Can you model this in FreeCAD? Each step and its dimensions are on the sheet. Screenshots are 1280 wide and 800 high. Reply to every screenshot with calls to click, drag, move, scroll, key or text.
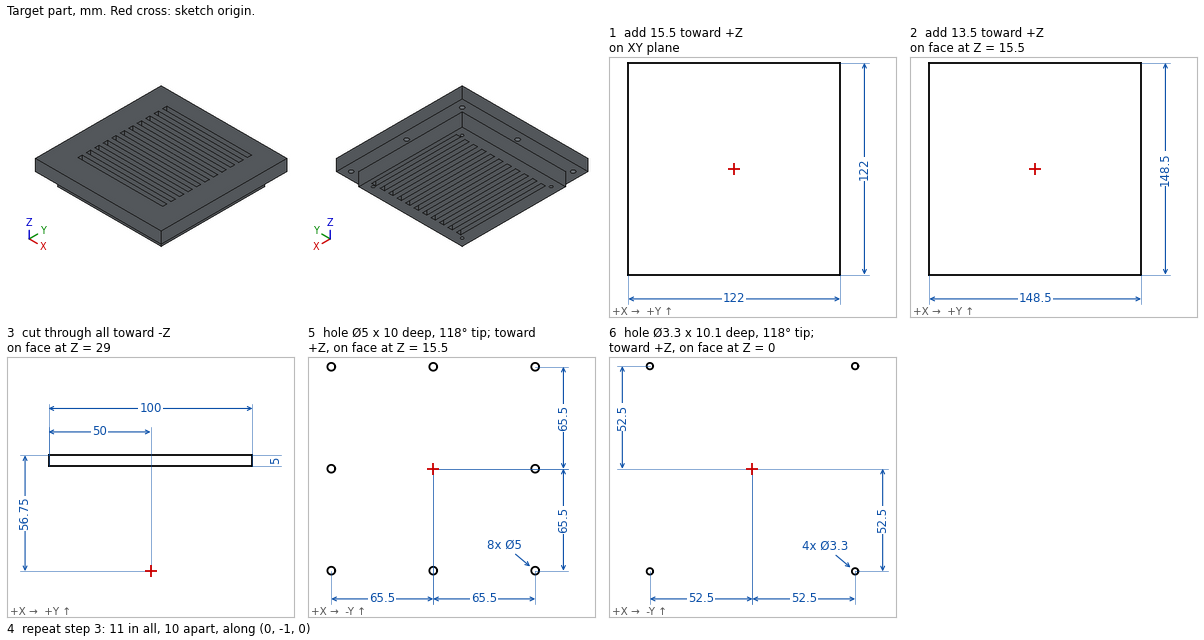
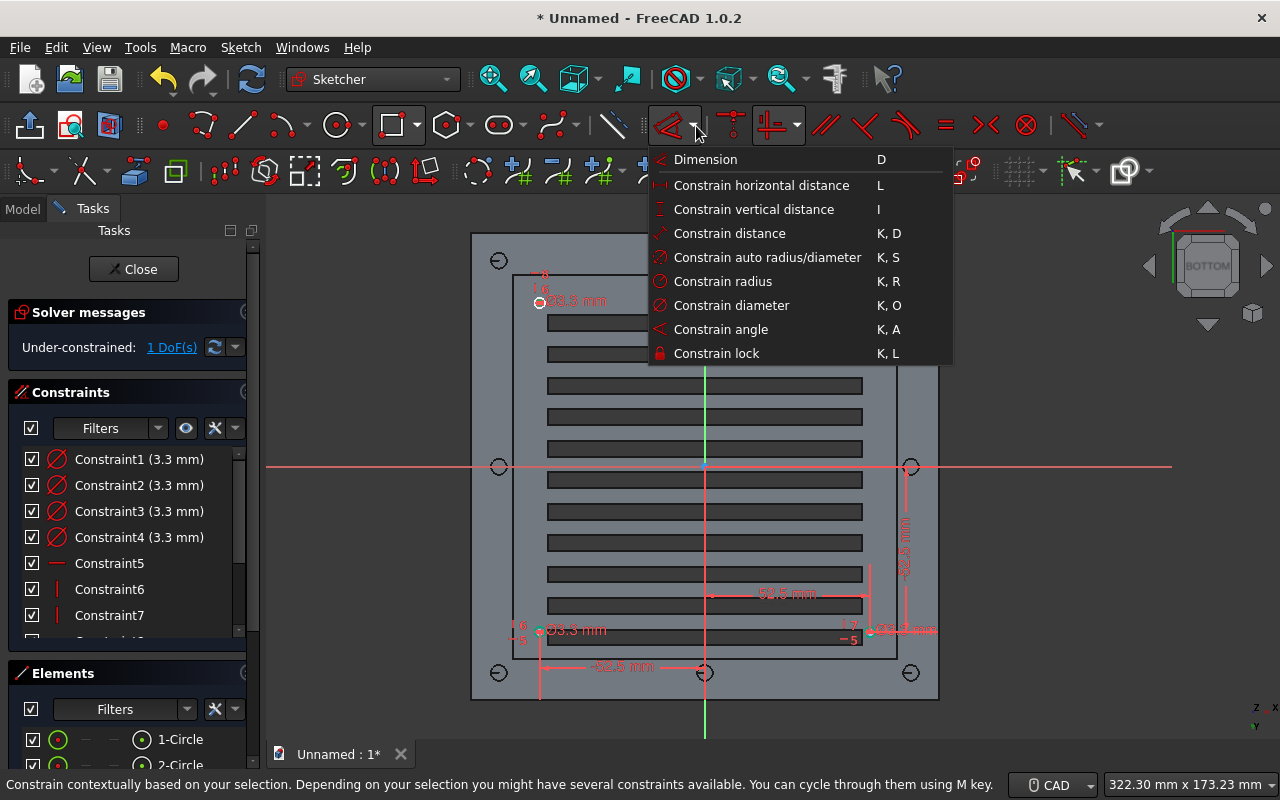
click(801, 209)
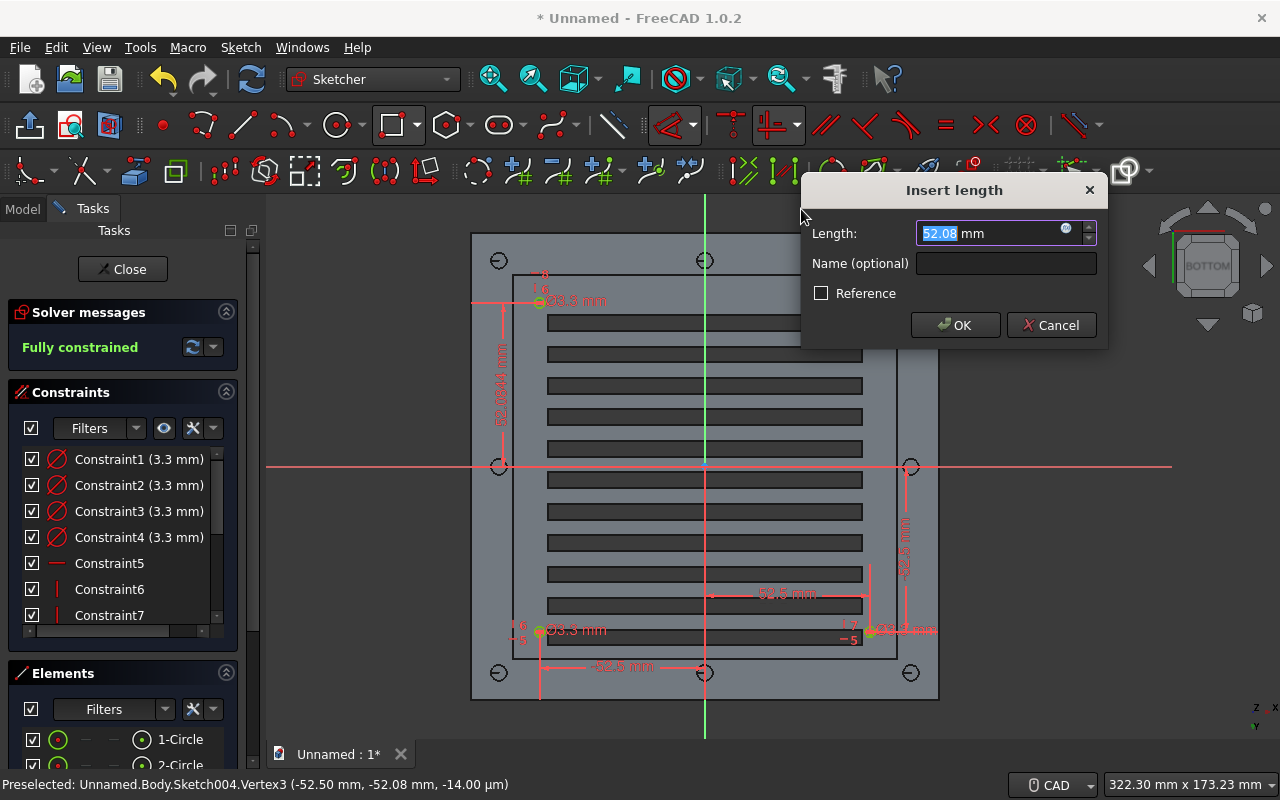
text(52.5)
key(Return)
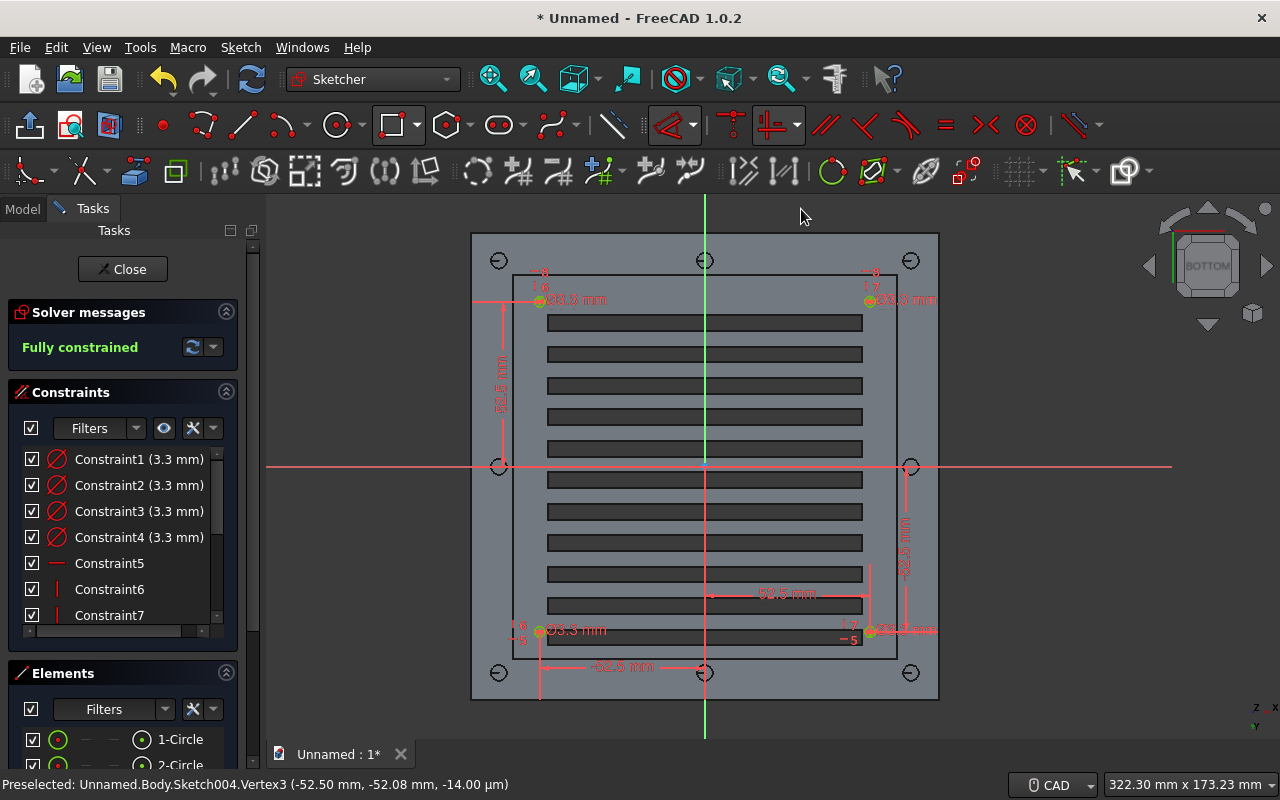
click(123, 269)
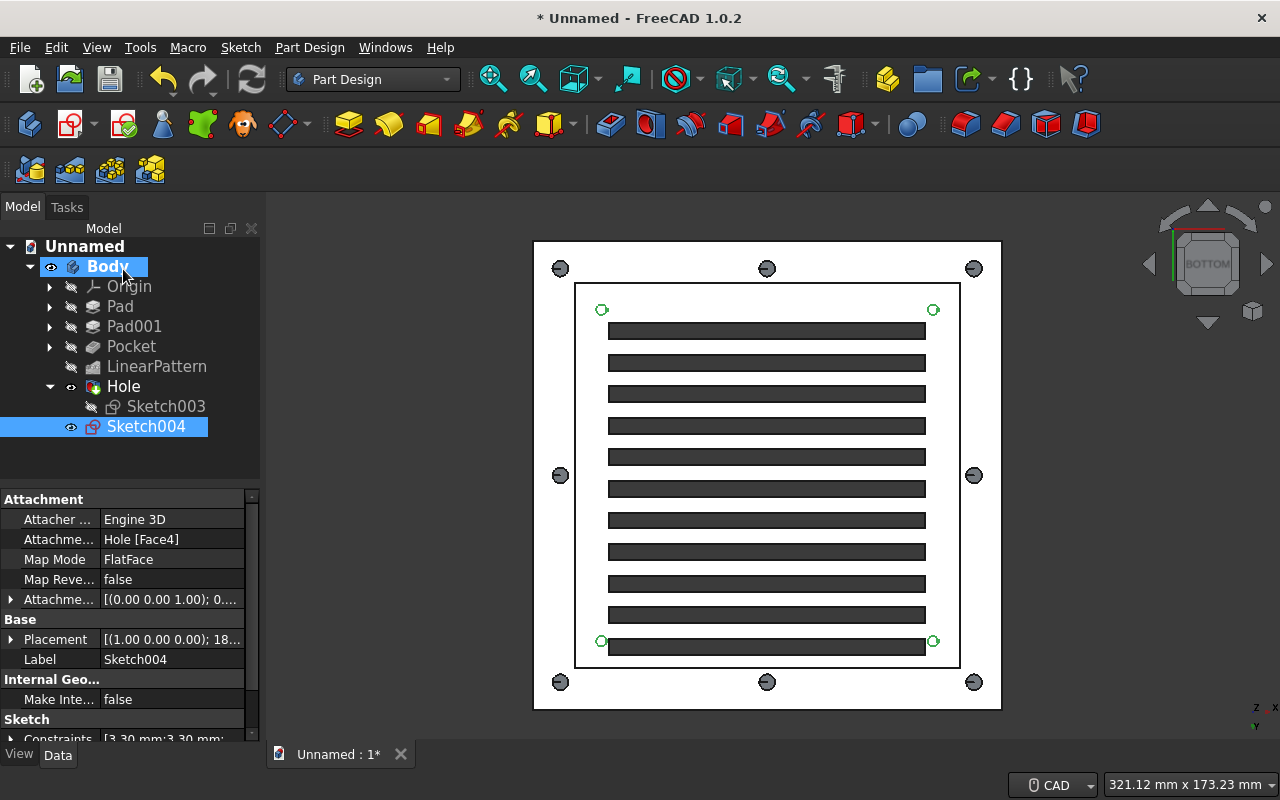
click(652, 124)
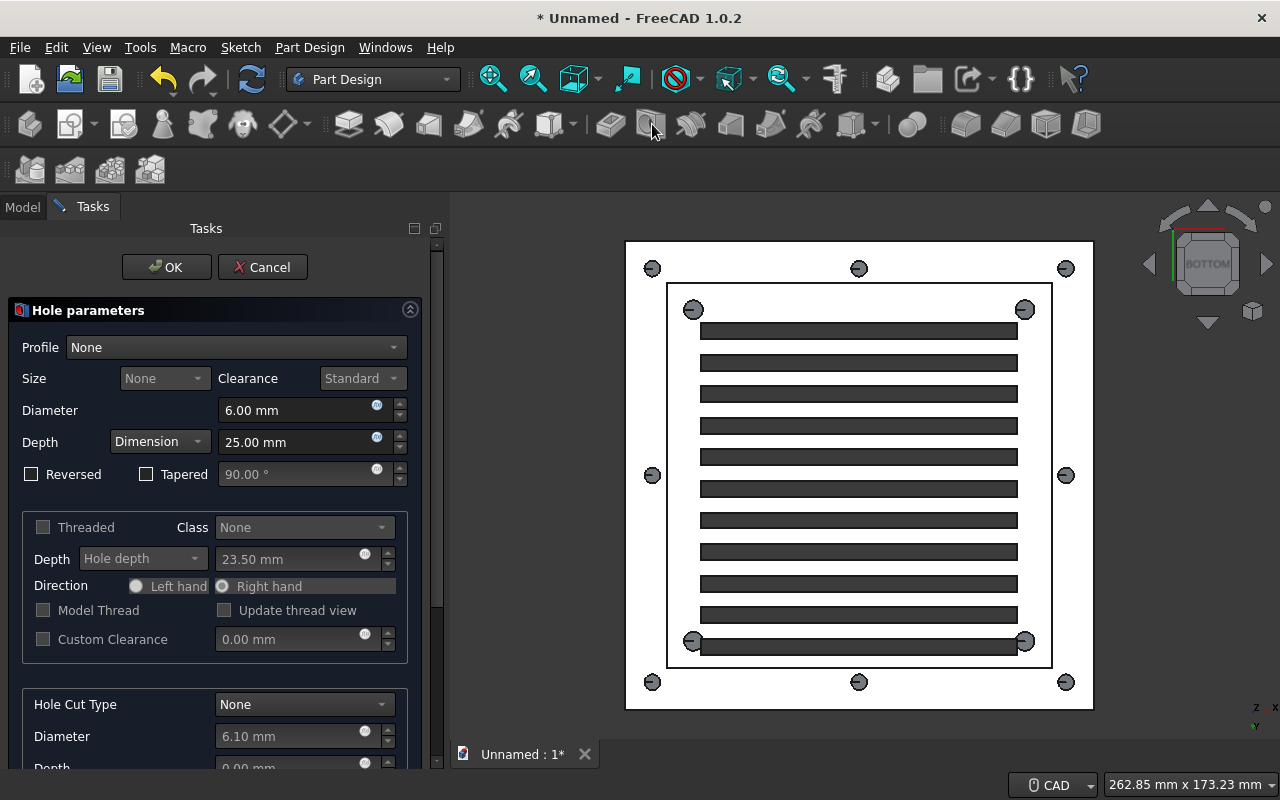
triple_click(305, 410)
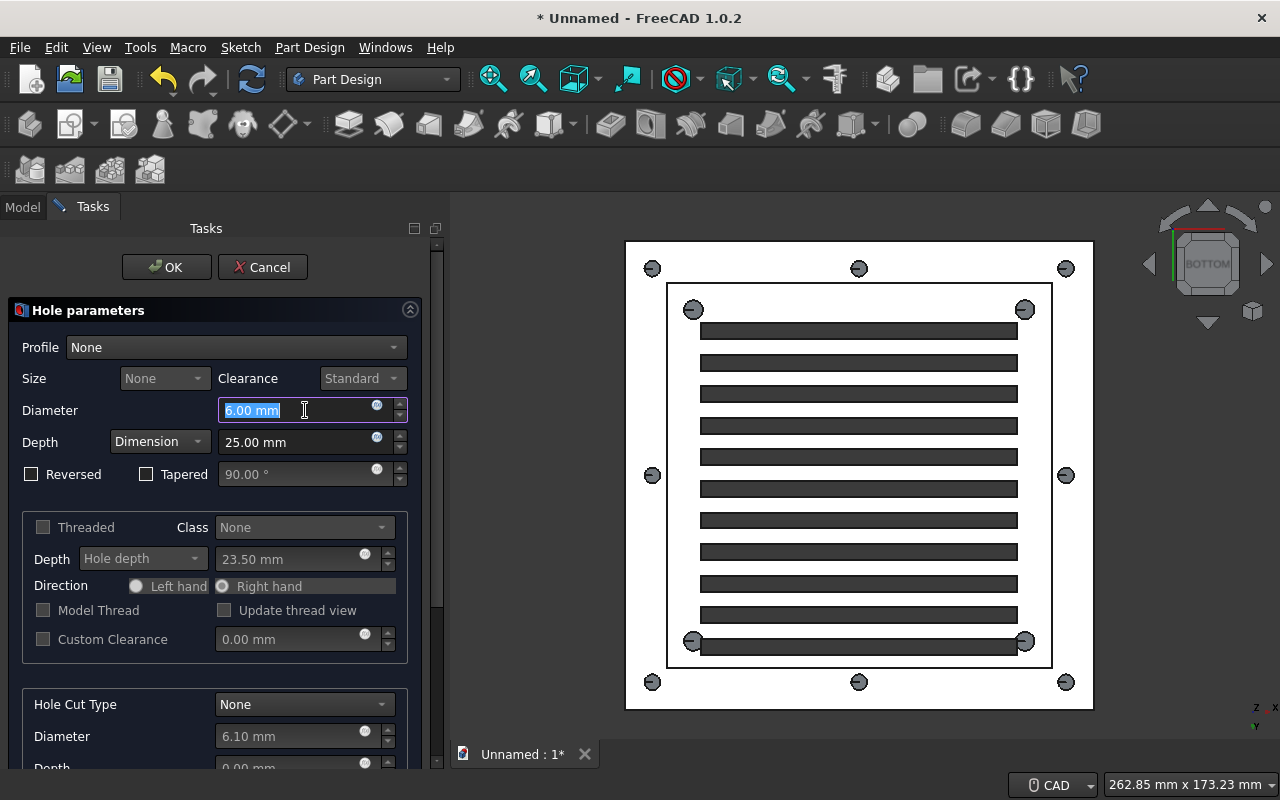
text(3.3)
key(Tab)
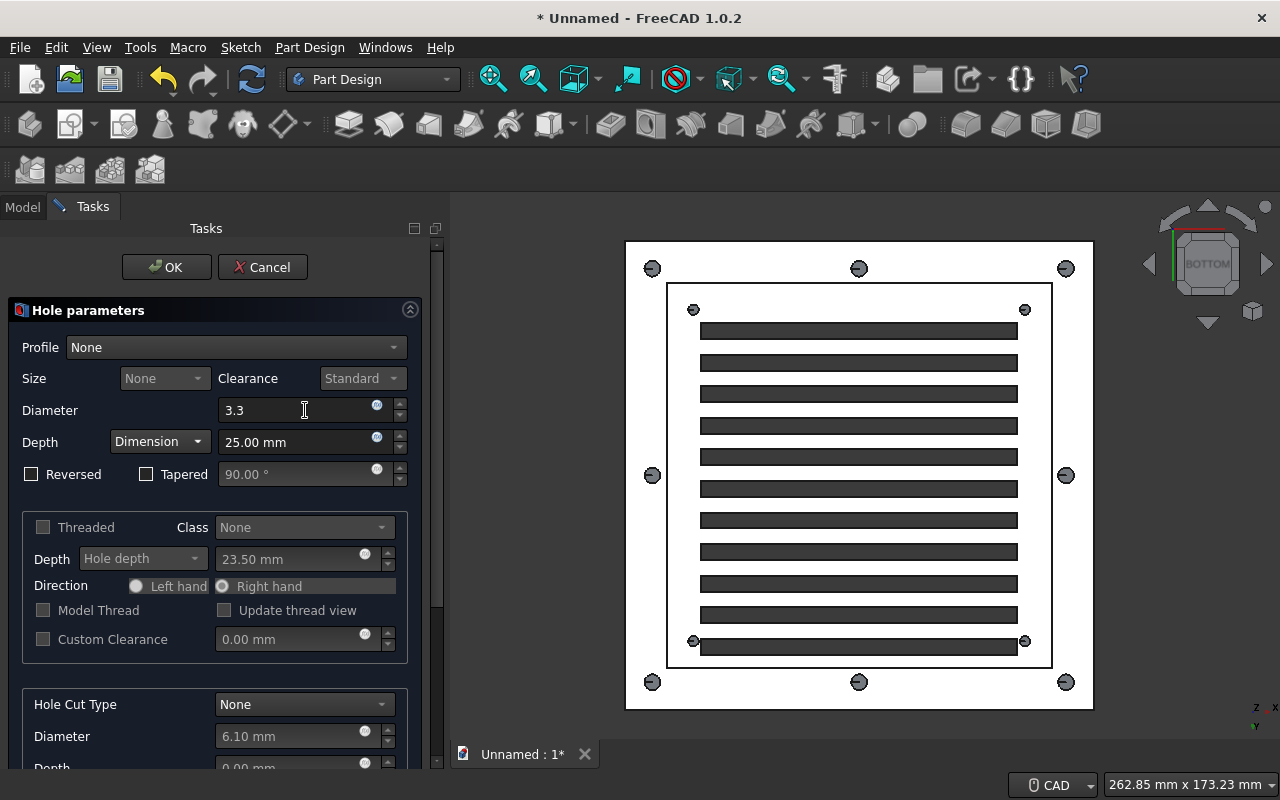
triple_click(305, 442)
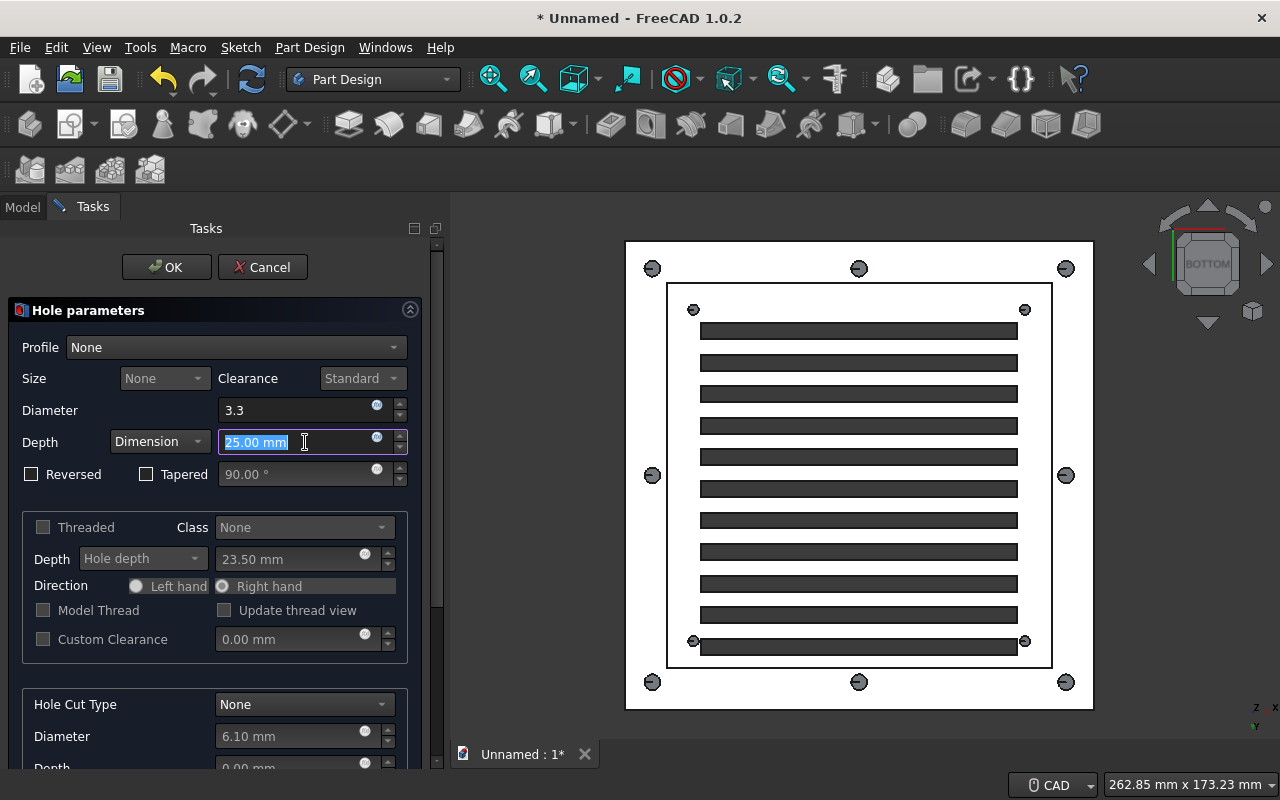
text(10.1)
key(Tab)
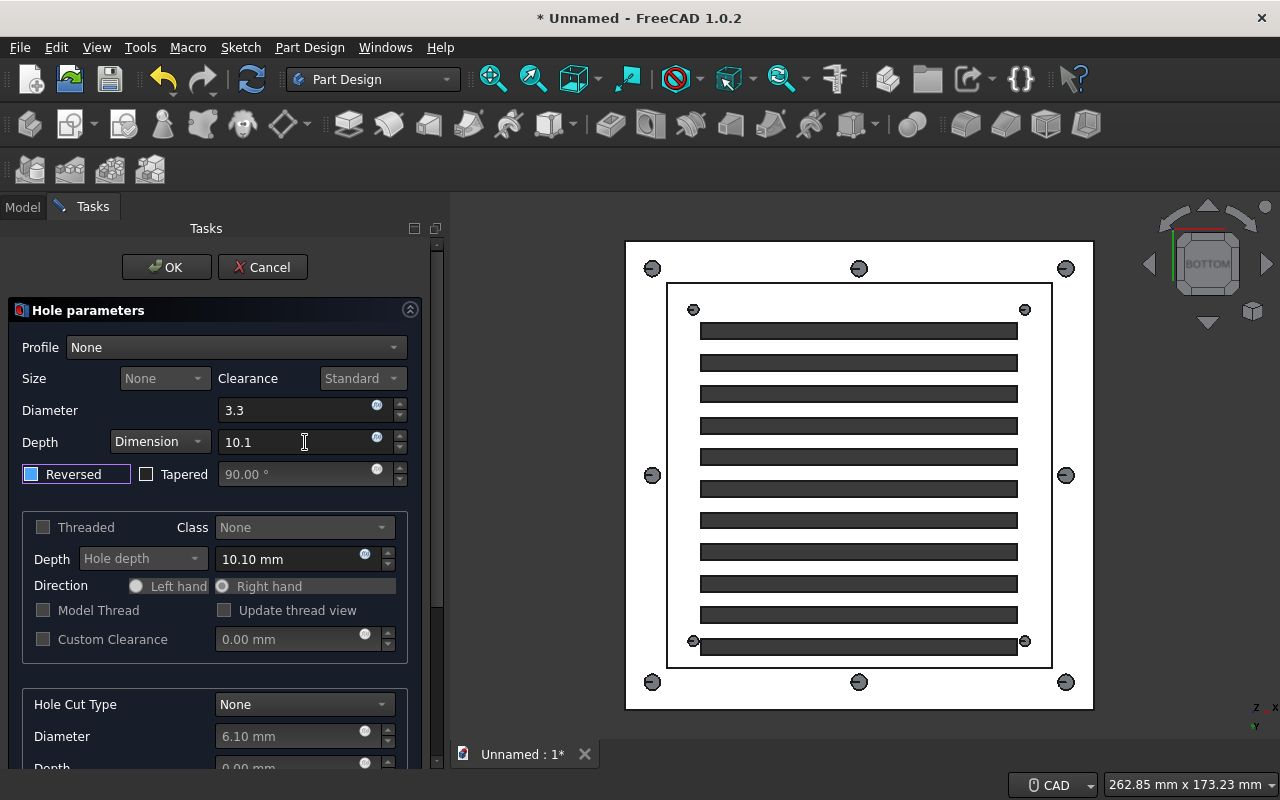
click(167, 267)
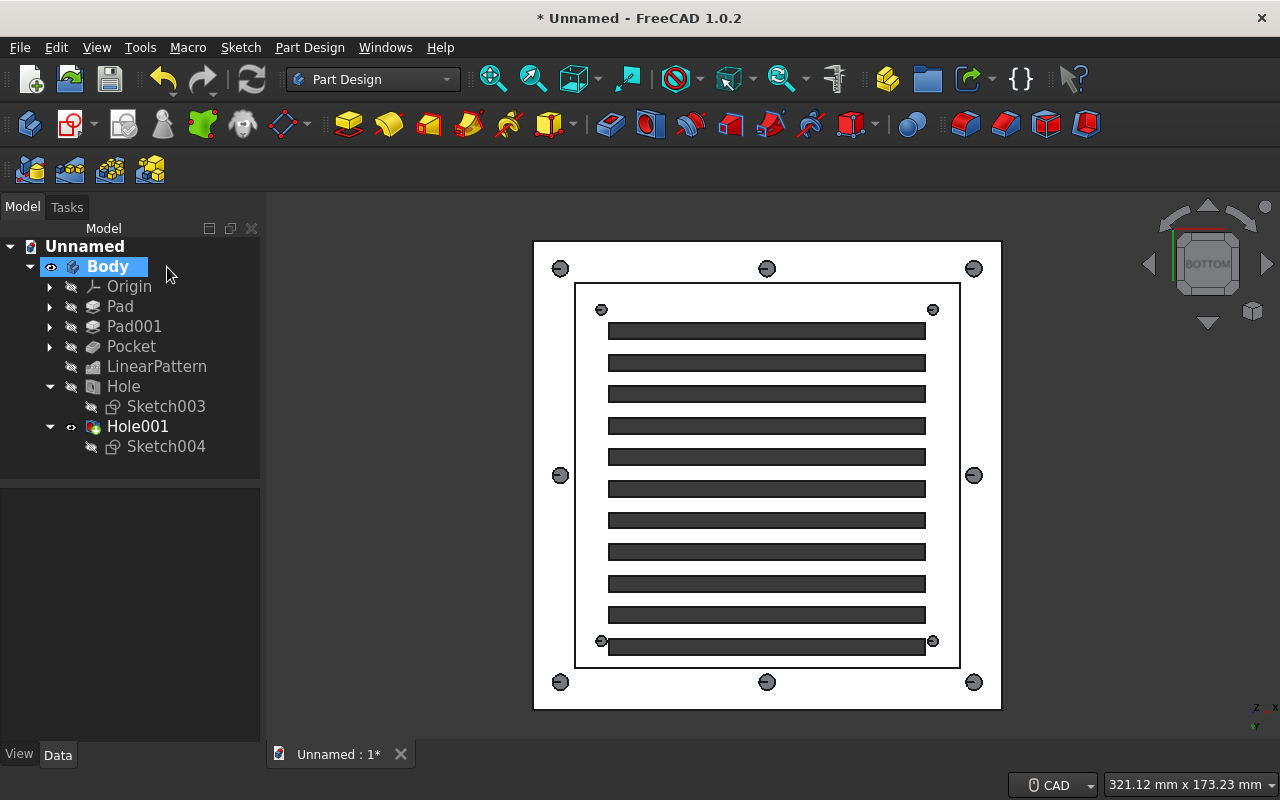
key(0)